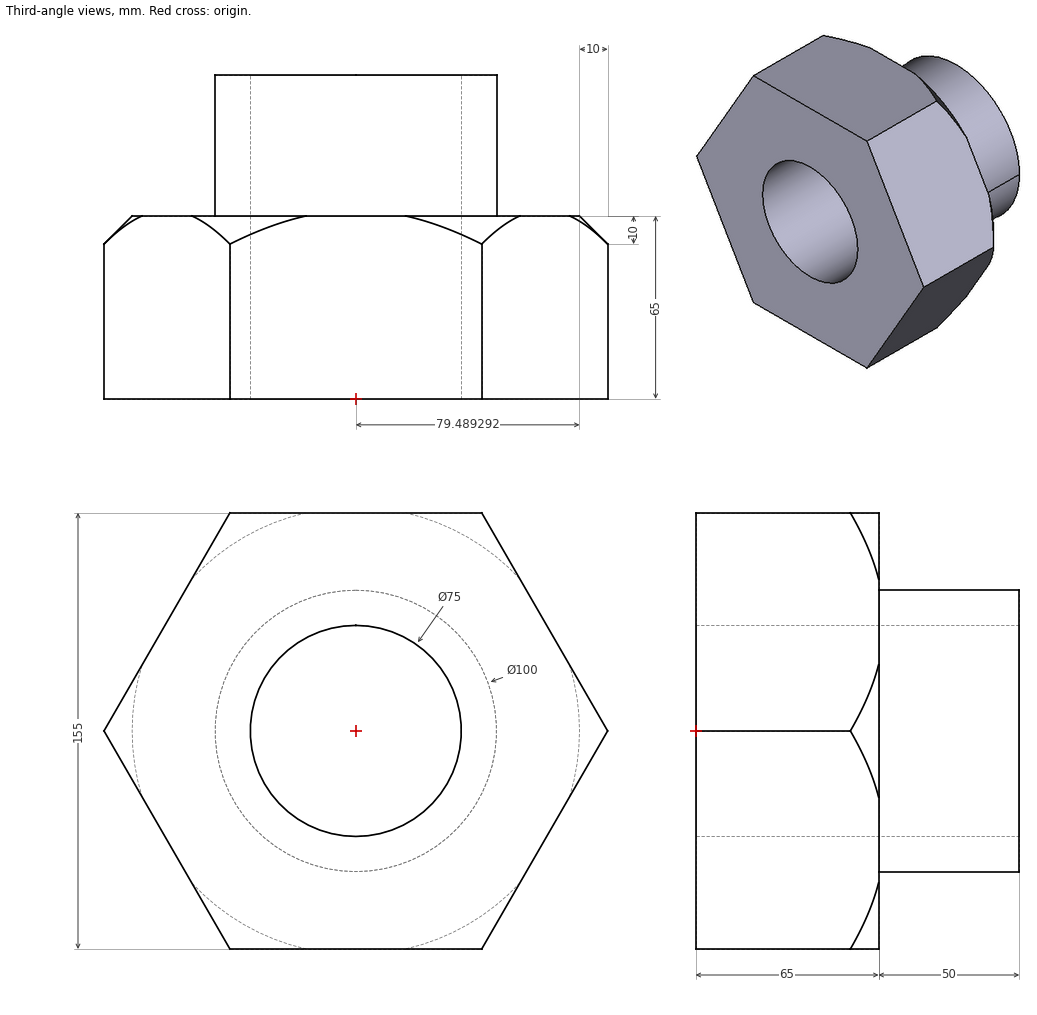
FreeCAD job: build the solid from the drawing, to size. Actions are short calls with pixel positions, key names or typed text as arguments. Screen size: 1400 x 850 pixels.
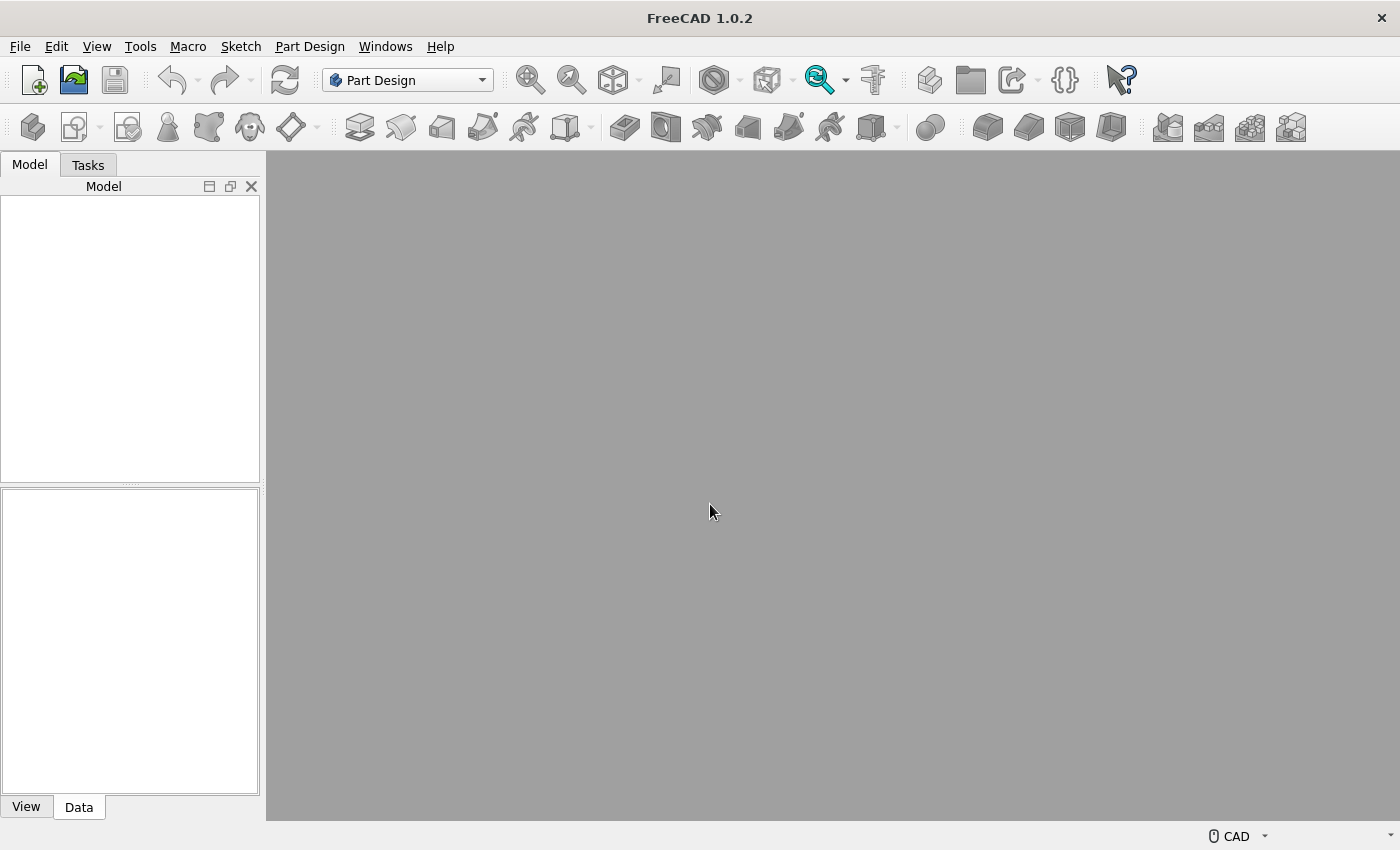
click(33, 80)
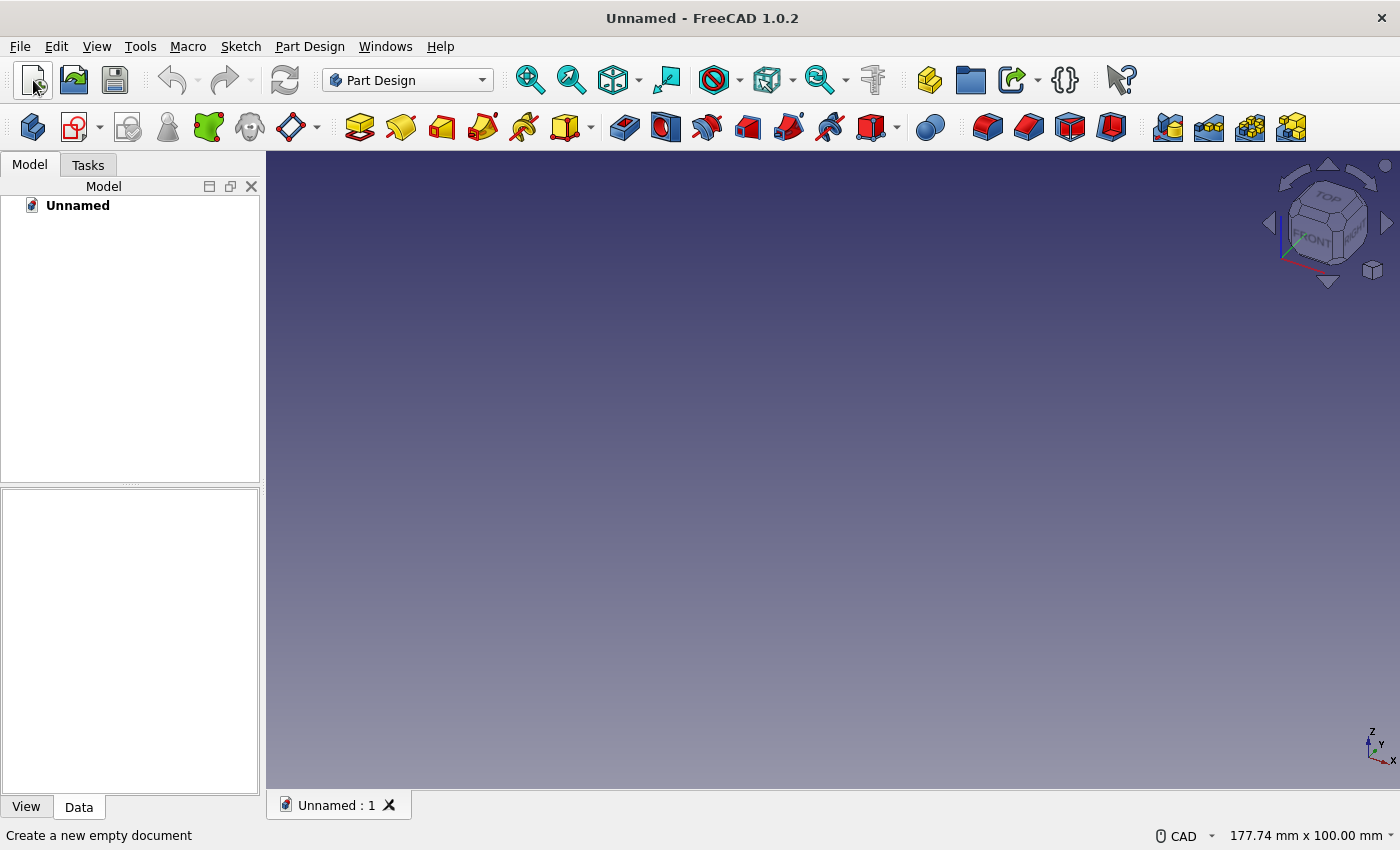
click(74, 128)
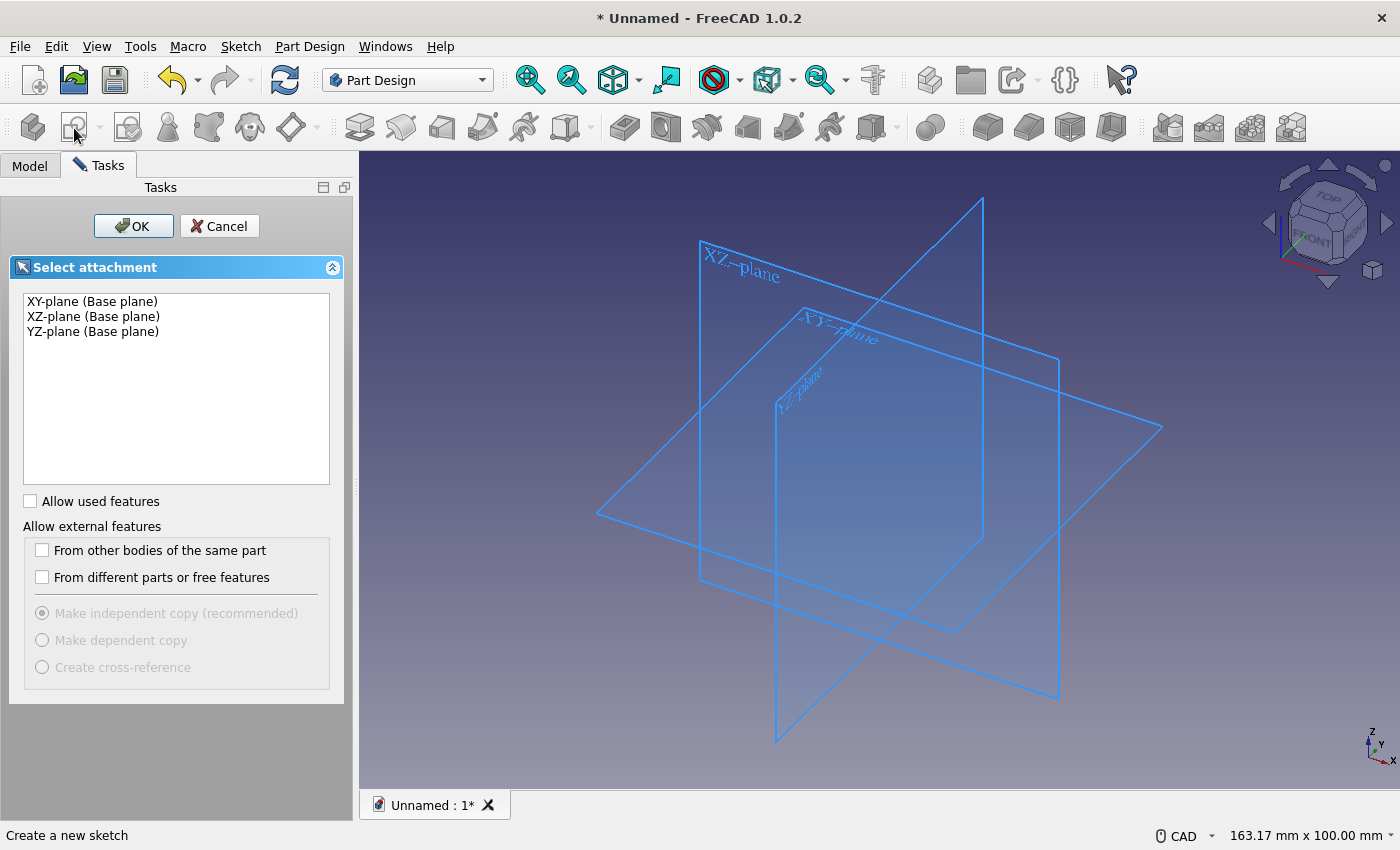
click(84, 316)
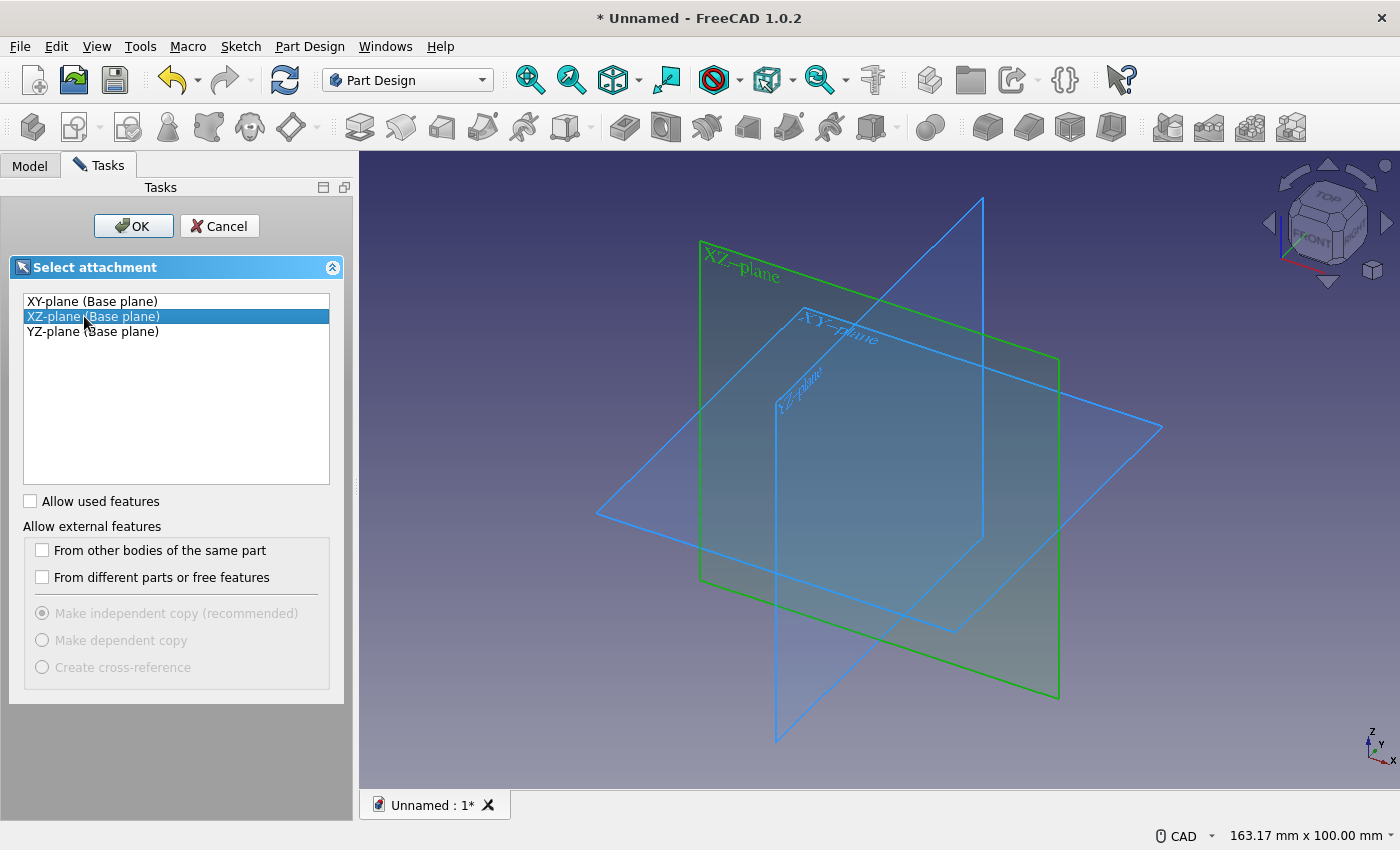
click(134, 226)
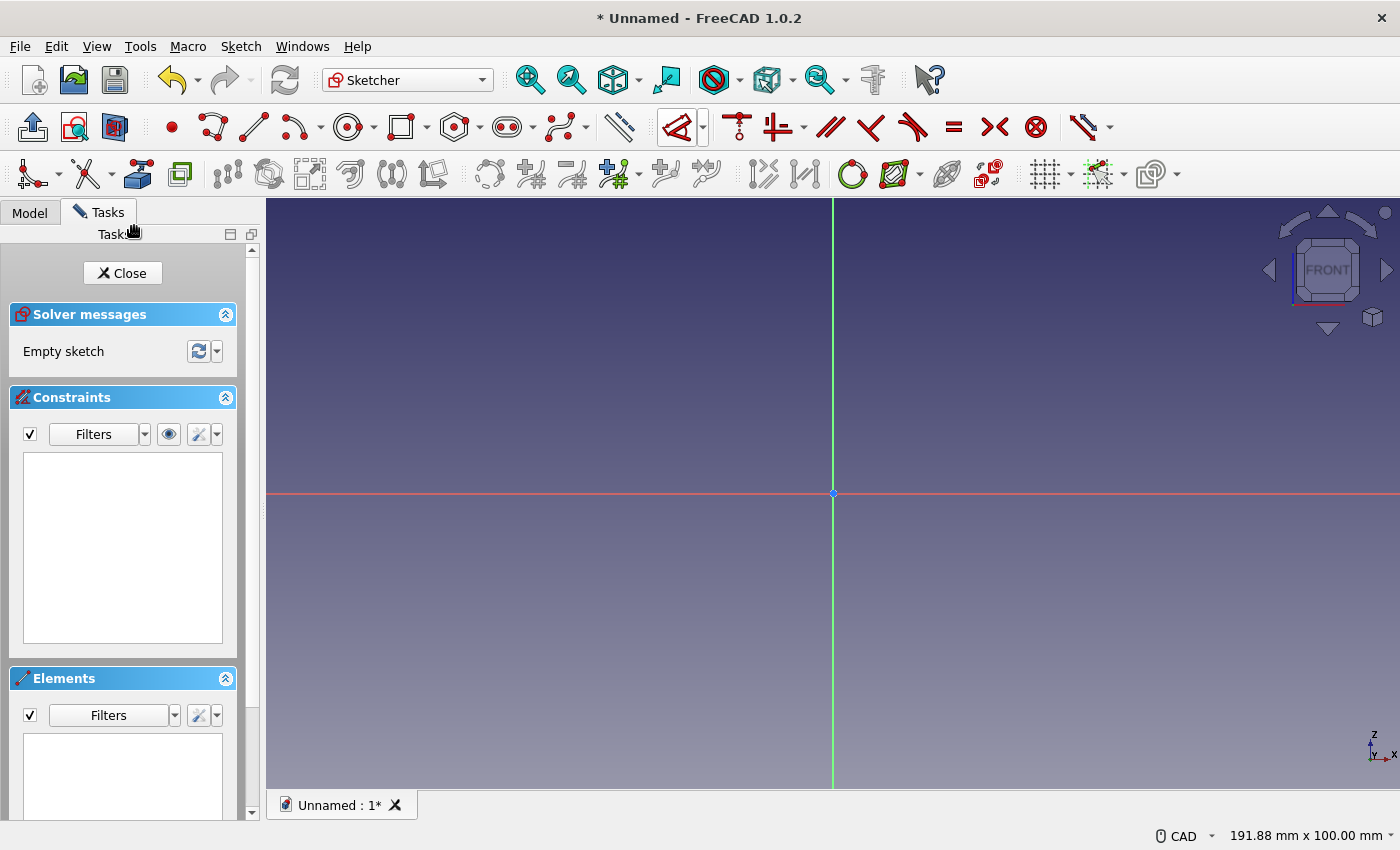
scroll(709, 494, down, 4)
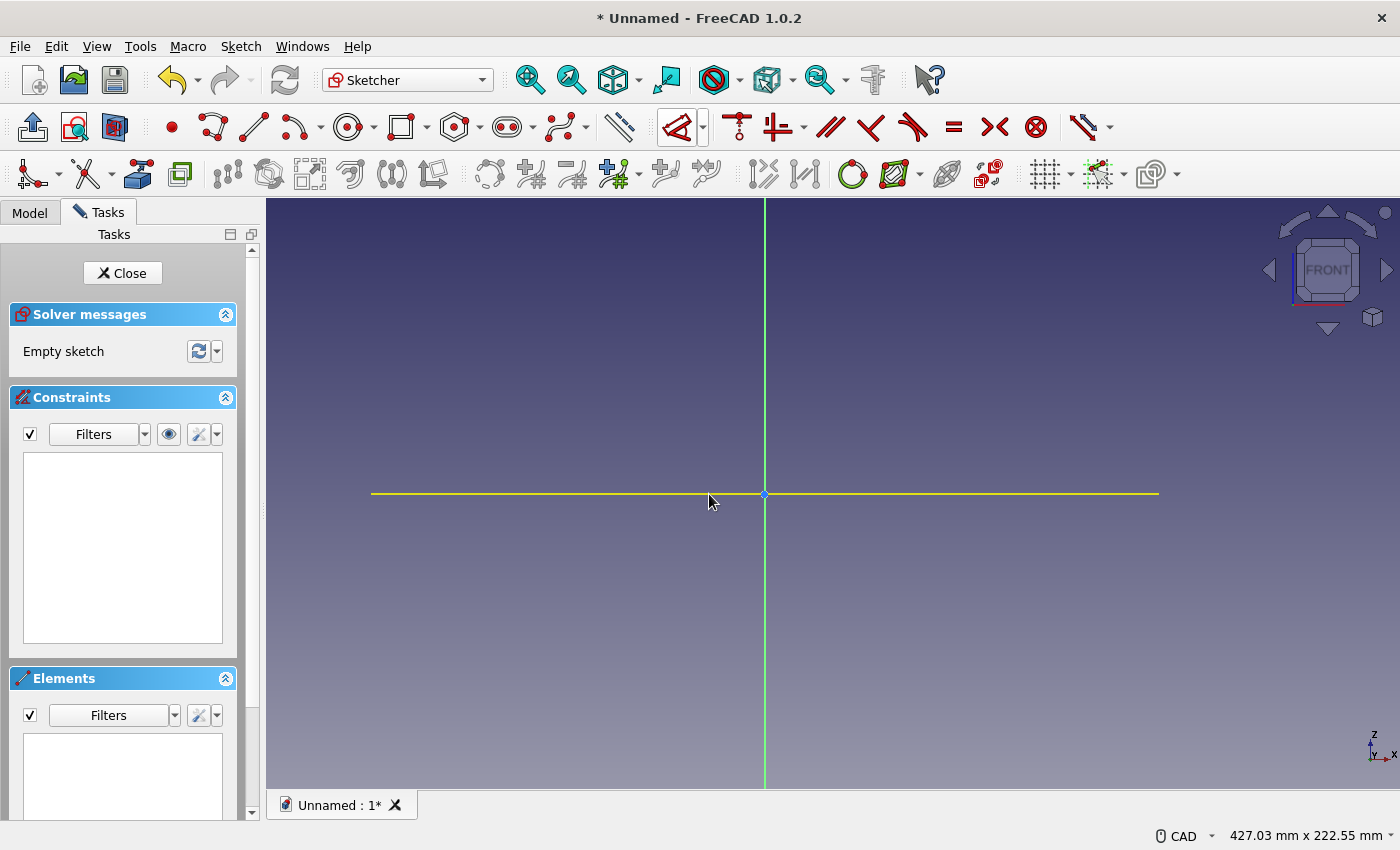
click(454, 128)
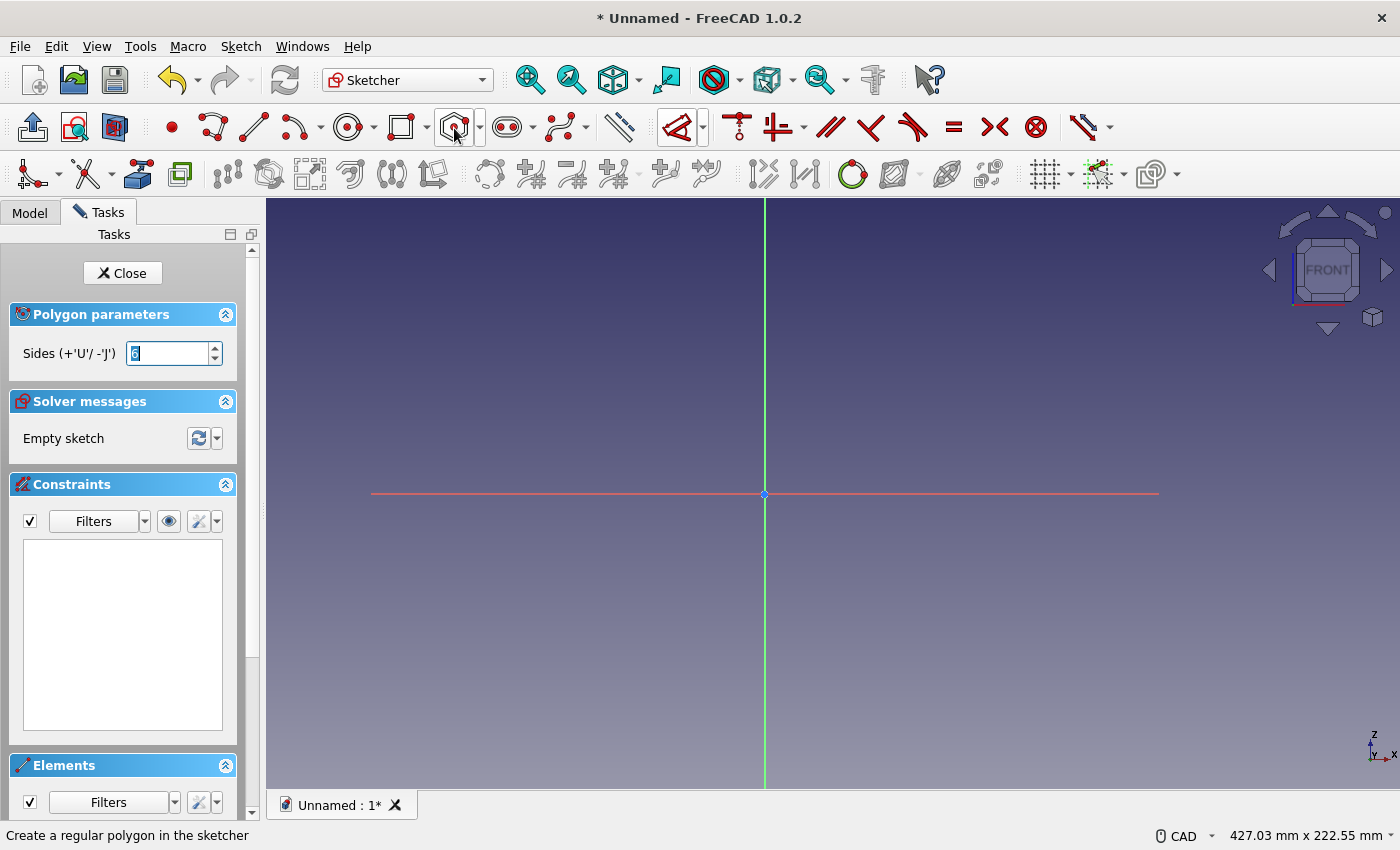
click(765, 494)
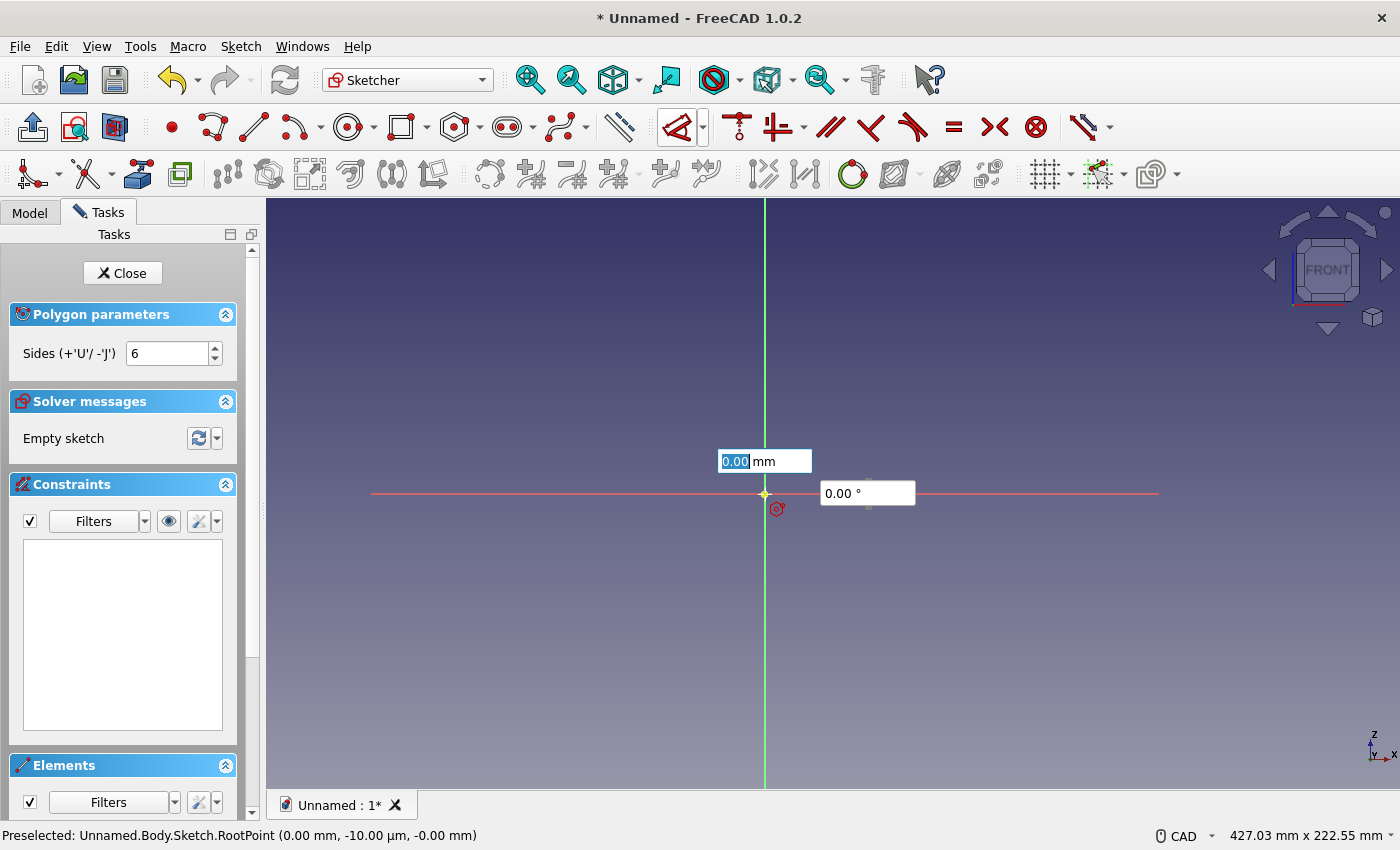
click(1003, 494)
right_click(1003, 494)